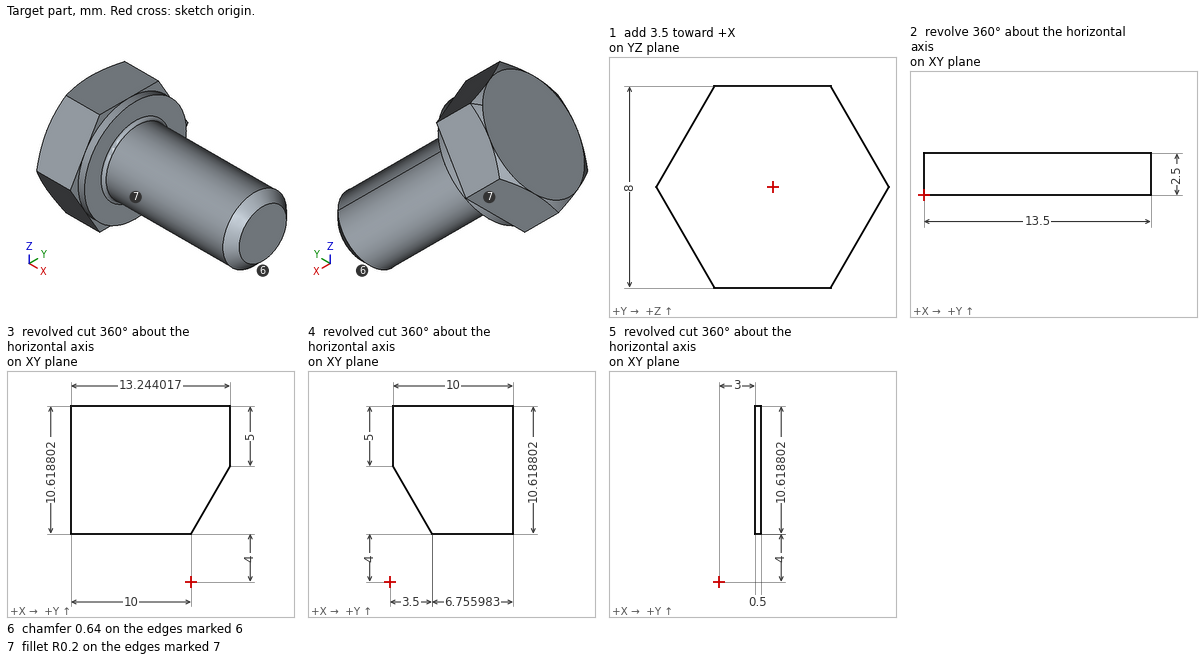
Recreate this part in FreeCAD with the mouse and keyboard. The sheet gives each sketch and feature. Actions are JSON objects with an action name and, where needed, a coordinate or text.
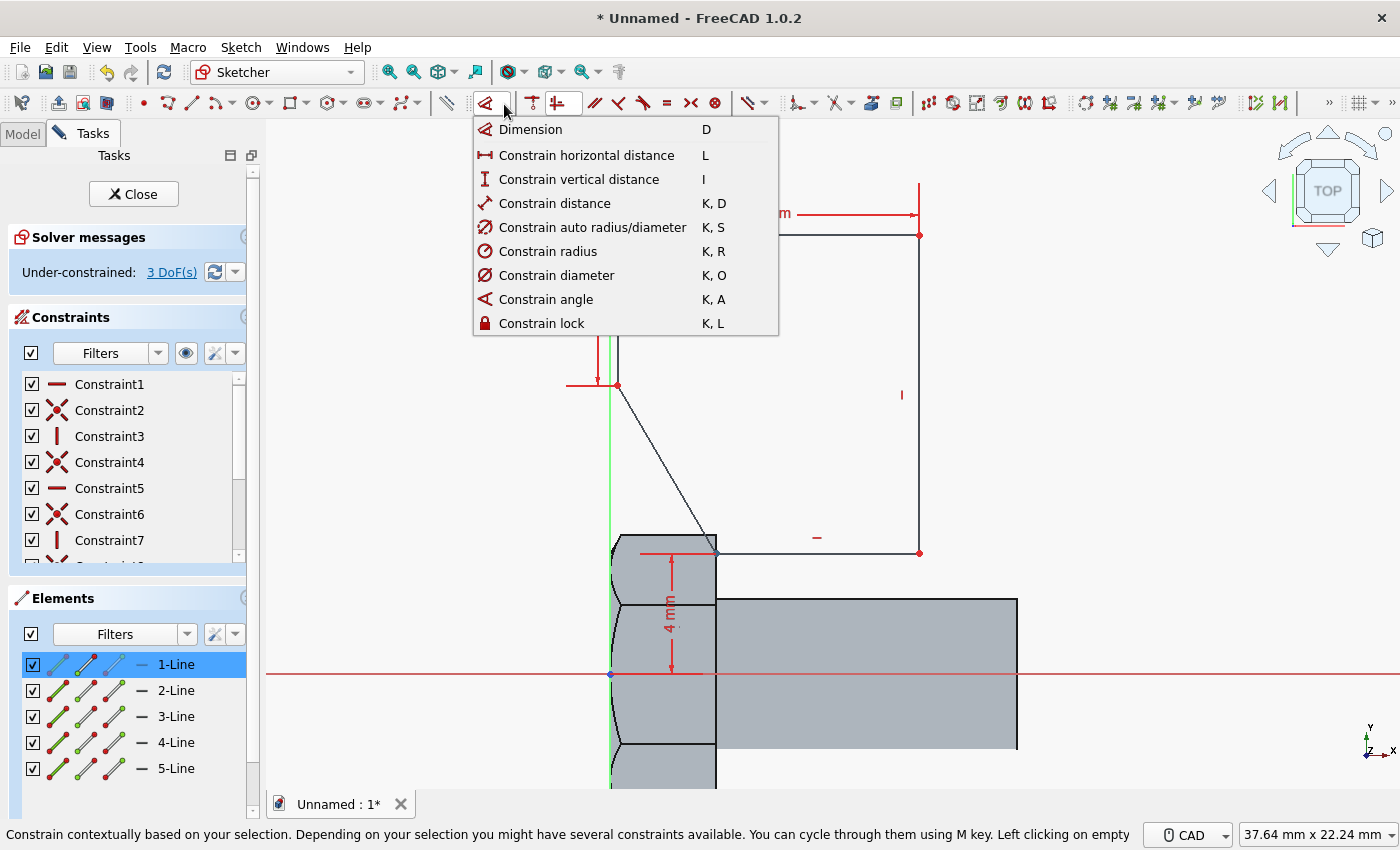
{"action": "left_click", "coordinate": [626, 155]}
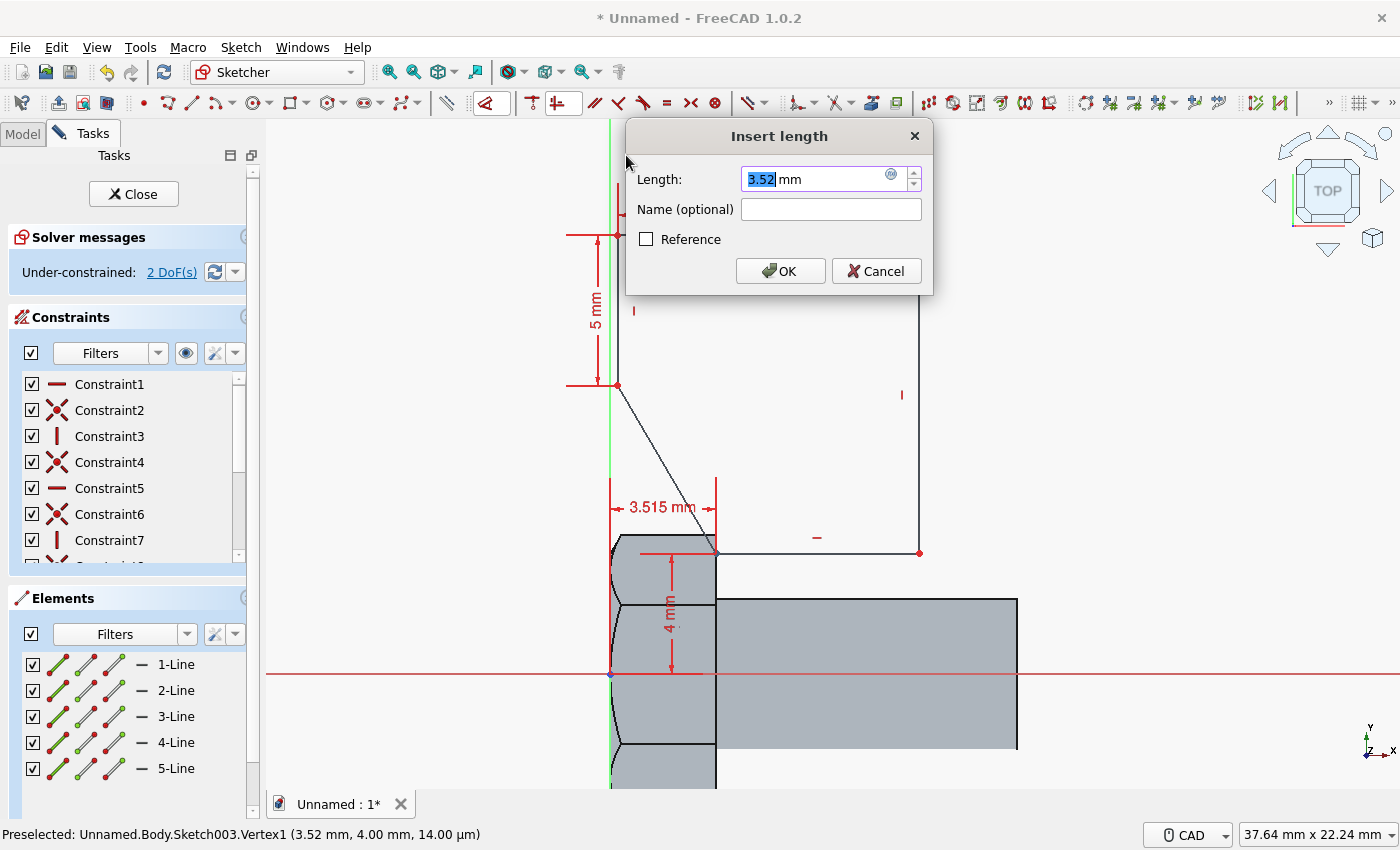
{"action": "type", "text": "3.5"}
{"action": "key", "text": "Return"}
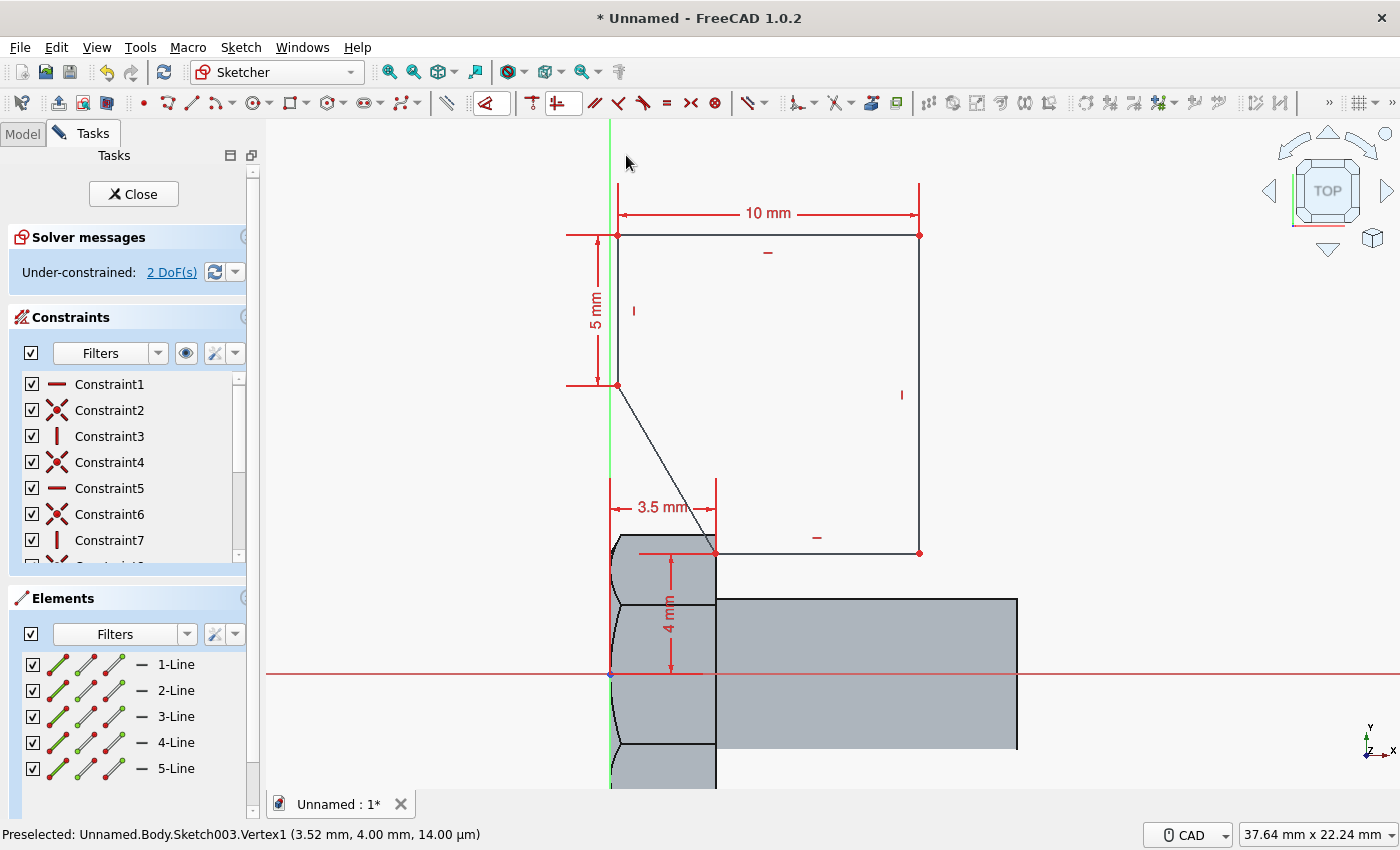
{"action": "left_click", "coordinate": [777, 554]}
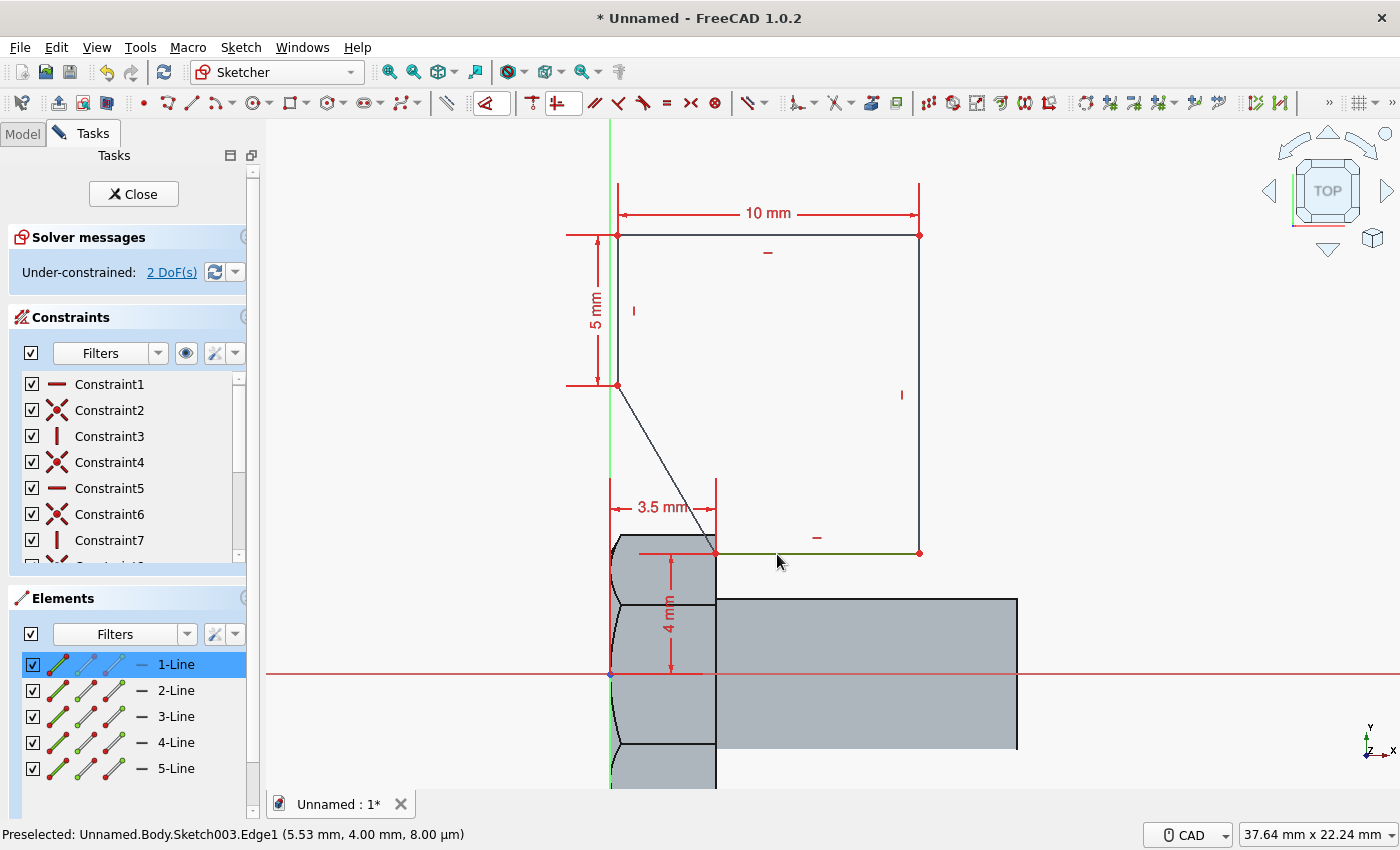
{"action": "left_click", "coordinate": [504, 104]}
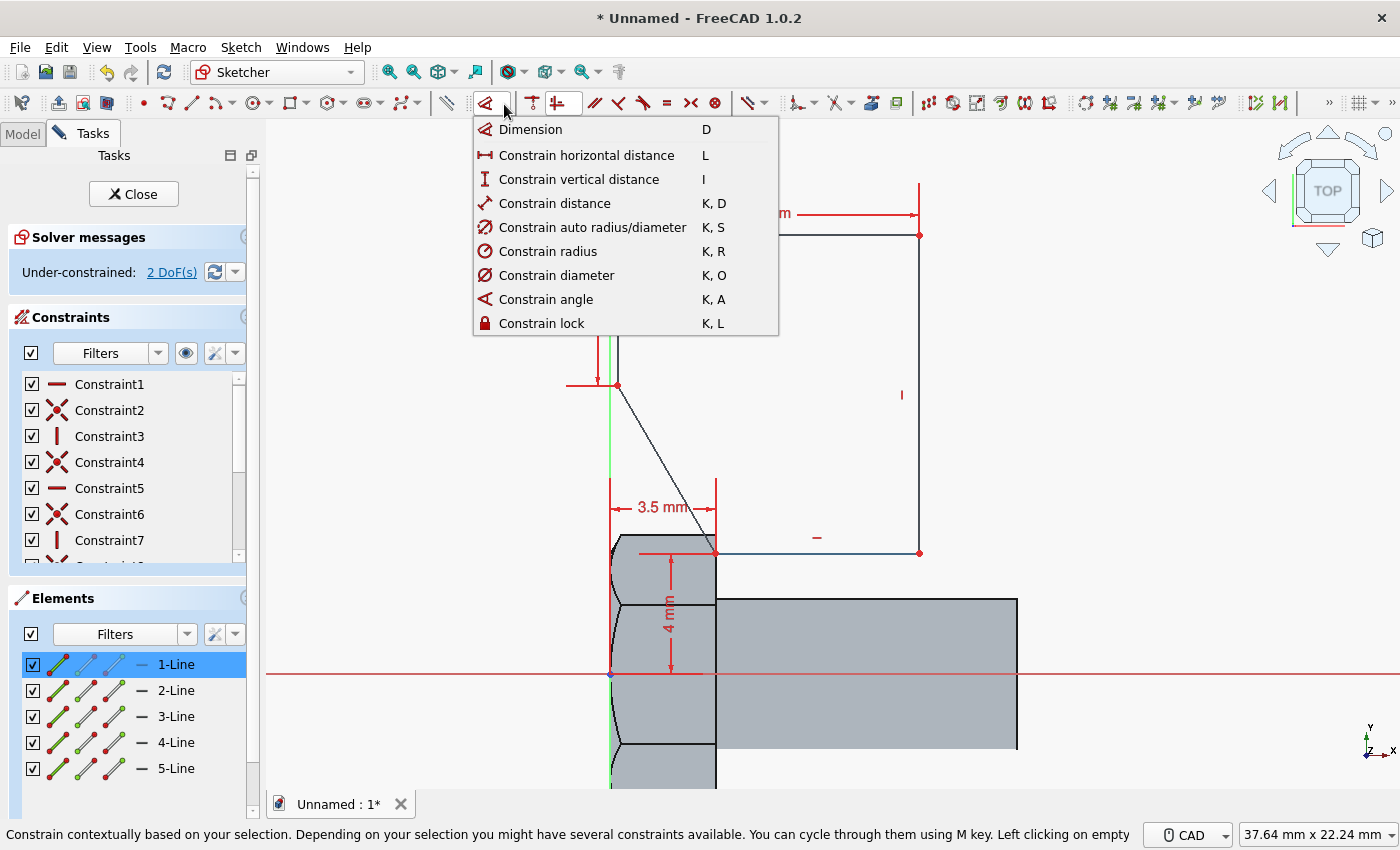
{"action": "left_click", "coordinate": [626, 155]}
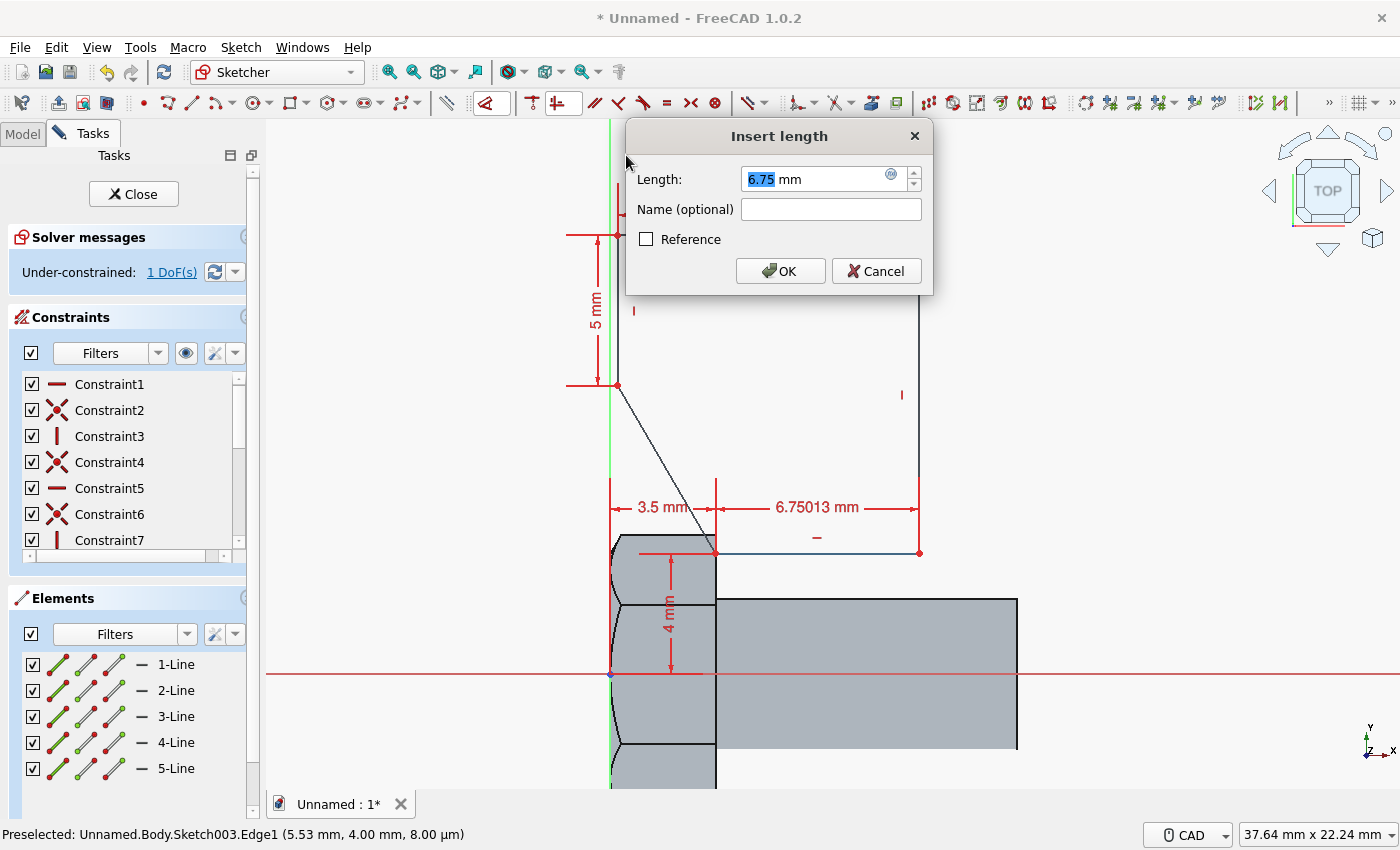
{"action": "type", "text": "6.755983"}
{"action": "key", "text": "Return"}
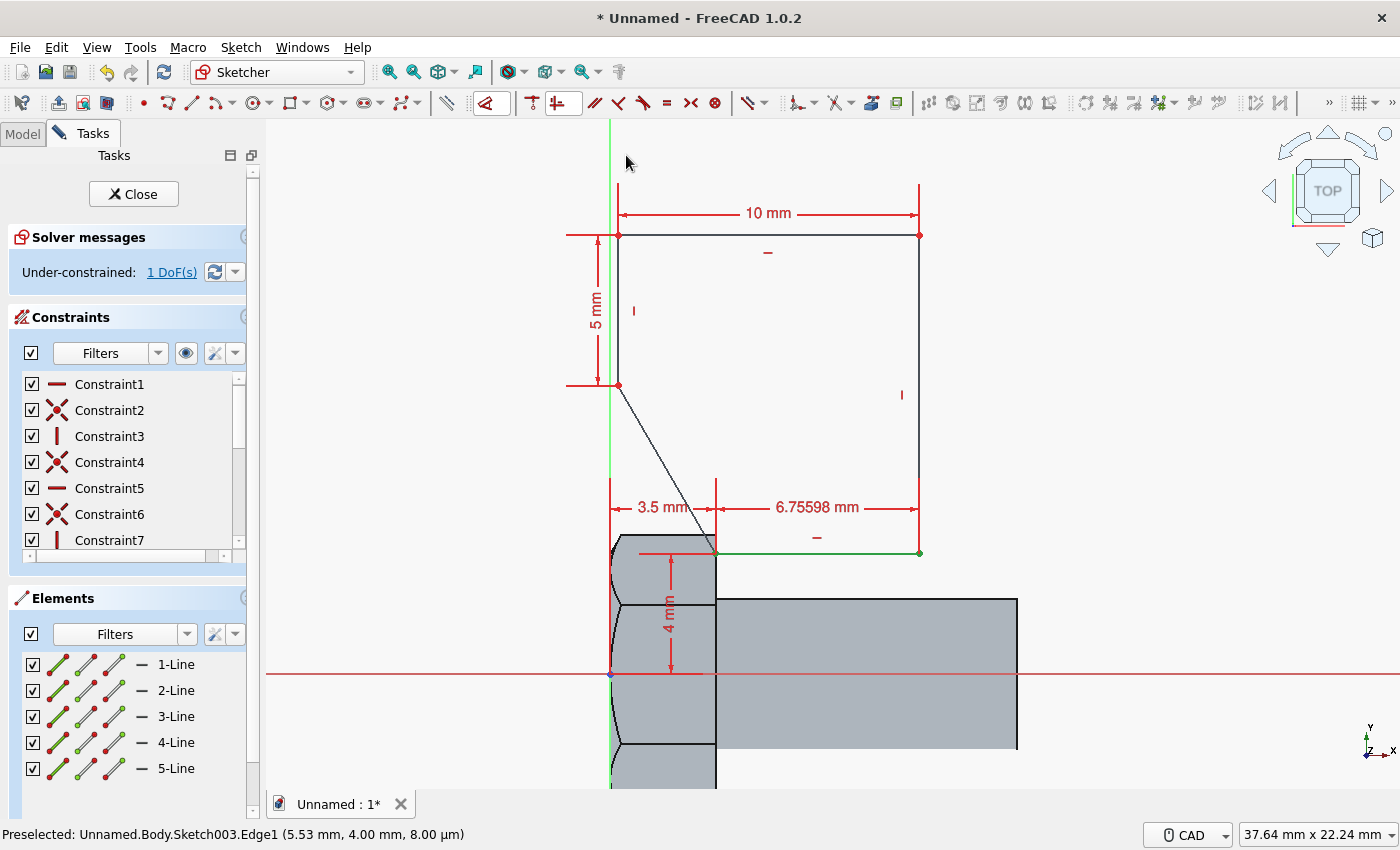
{"action": "left_click", "coordinate": [919, 458]}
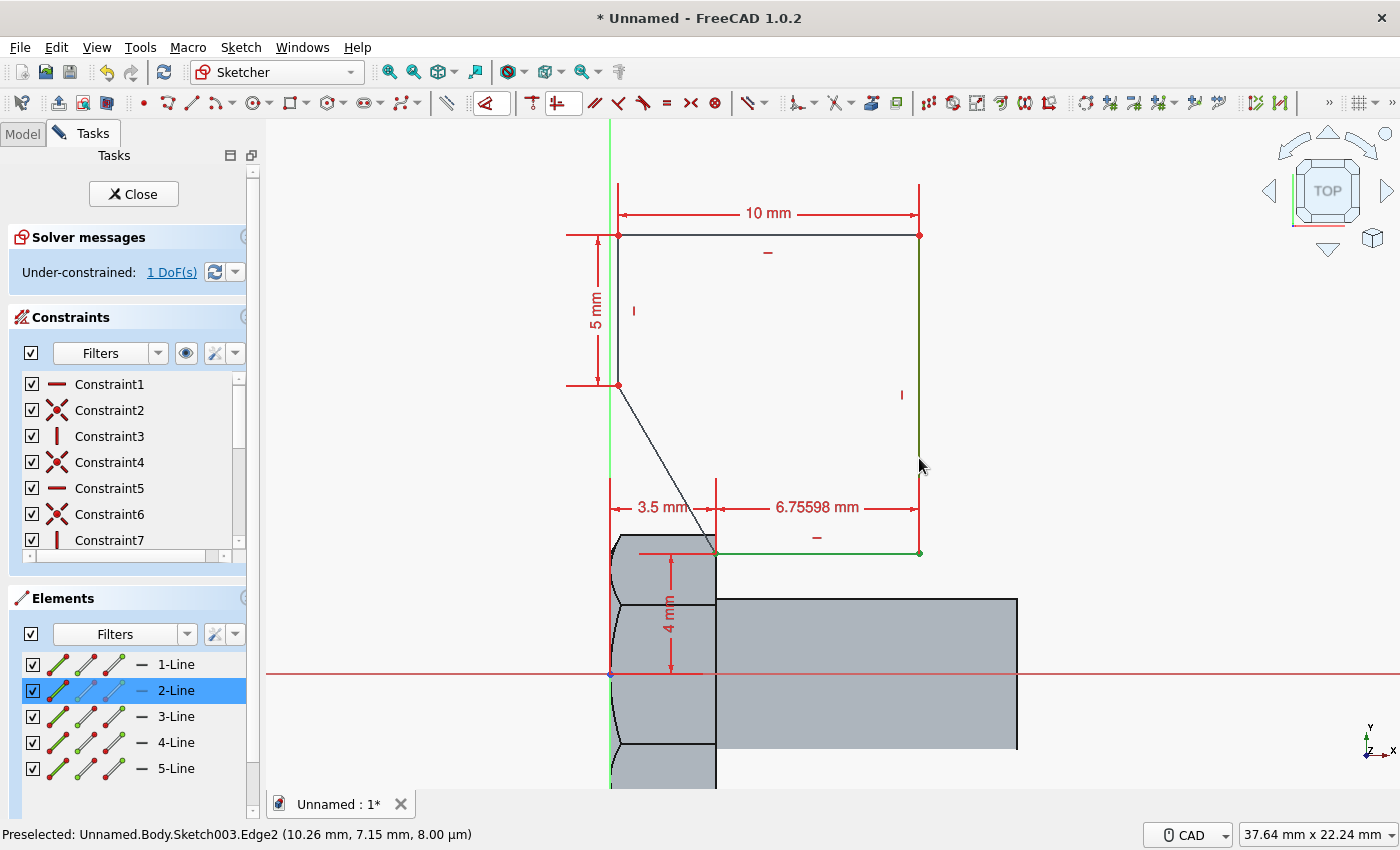
{"action": "left_click", "coordinate": [504, 104]}